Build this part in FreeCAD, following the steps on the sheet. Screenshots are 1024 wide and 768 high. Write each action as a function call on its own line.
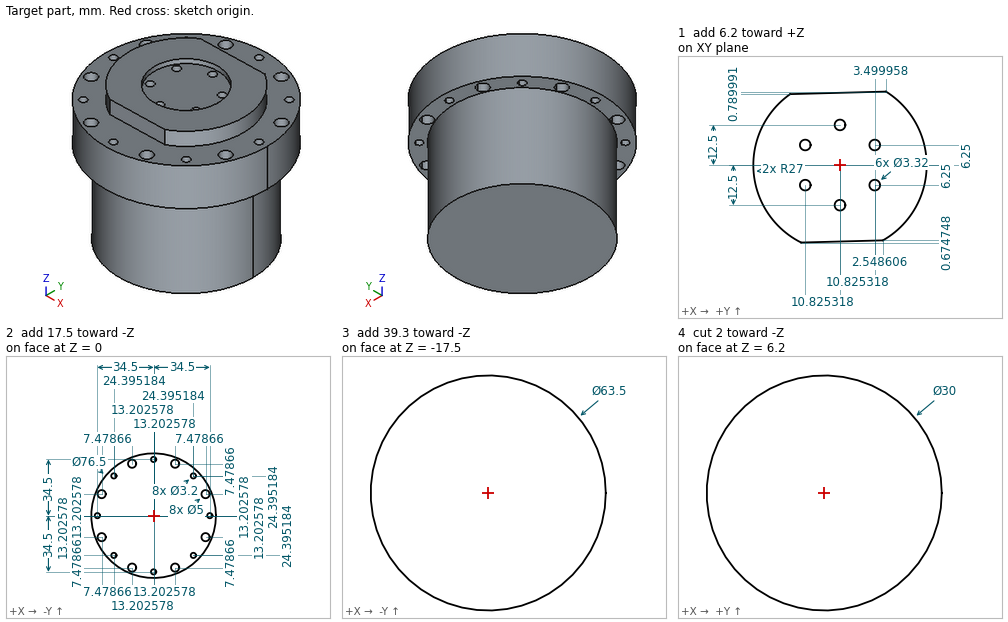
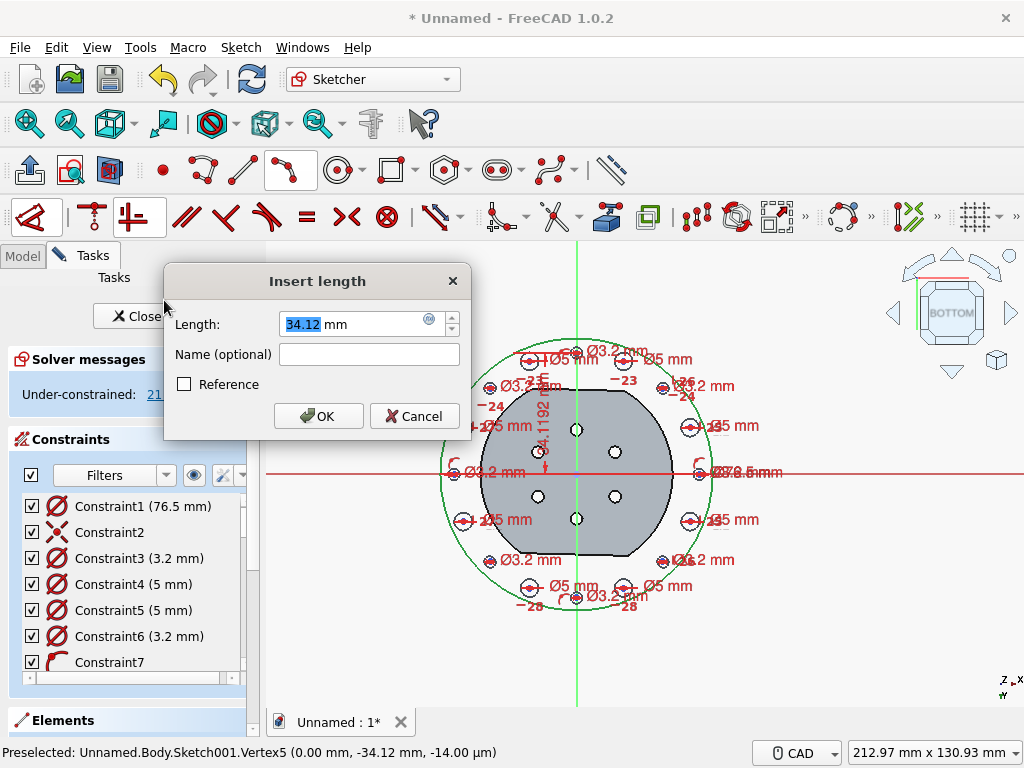
text(34.5)
key(Return)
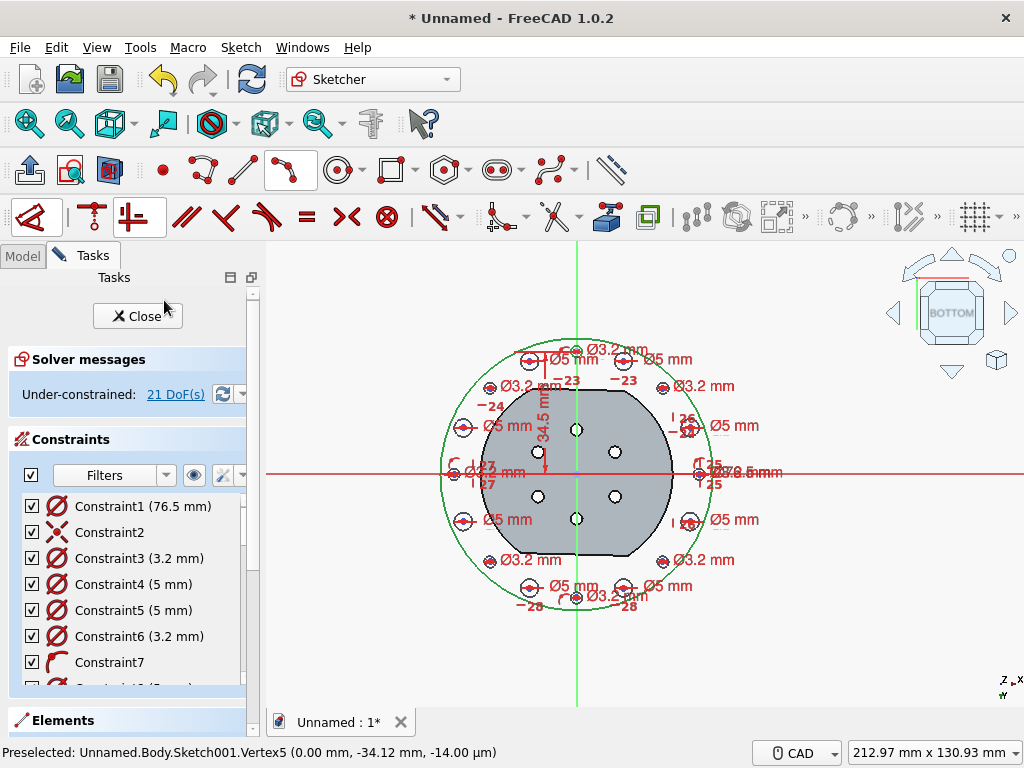
click(699, 474)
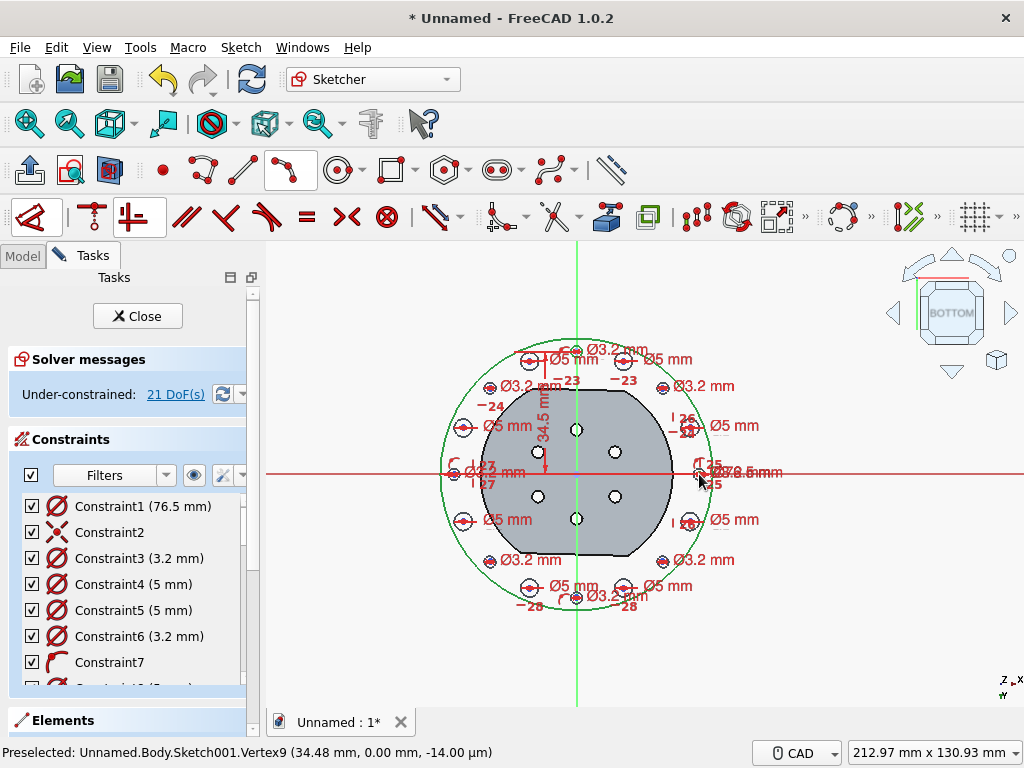
key(l)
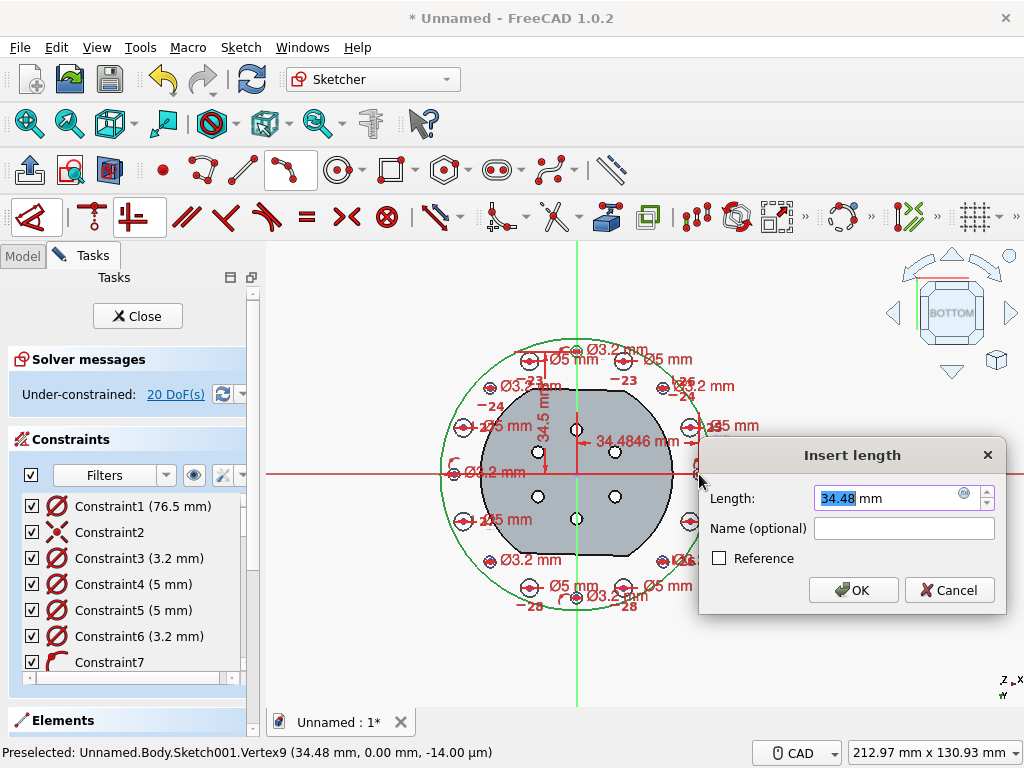
text(34.5)
key(Return)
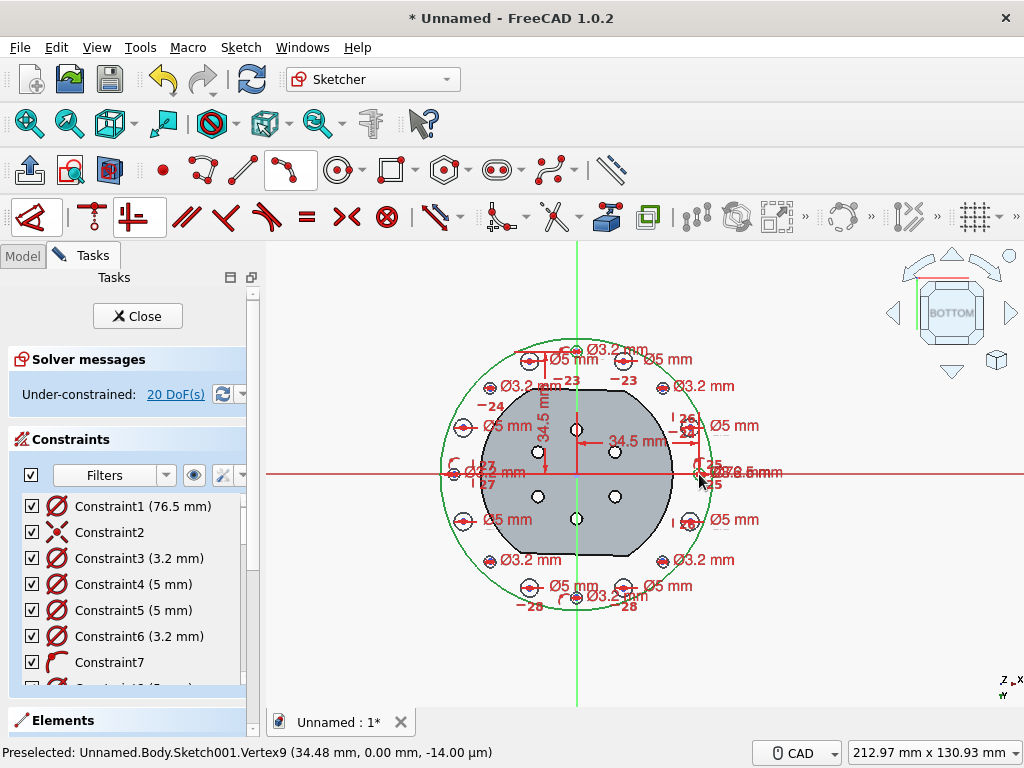
click(454, 474)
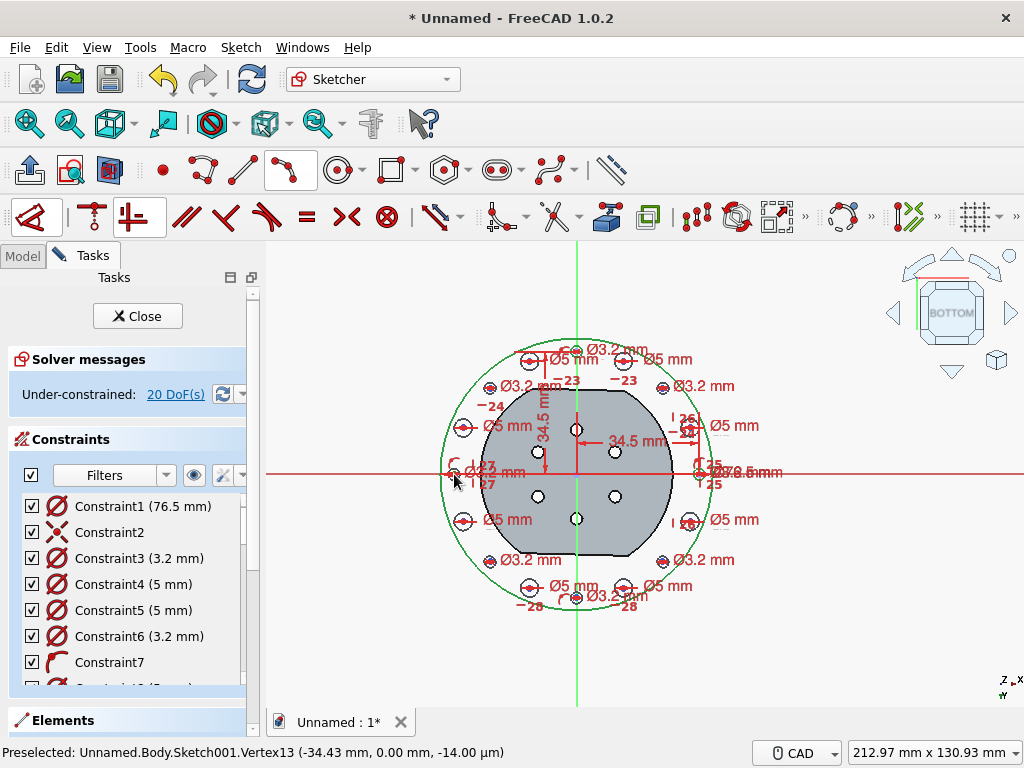
key(l)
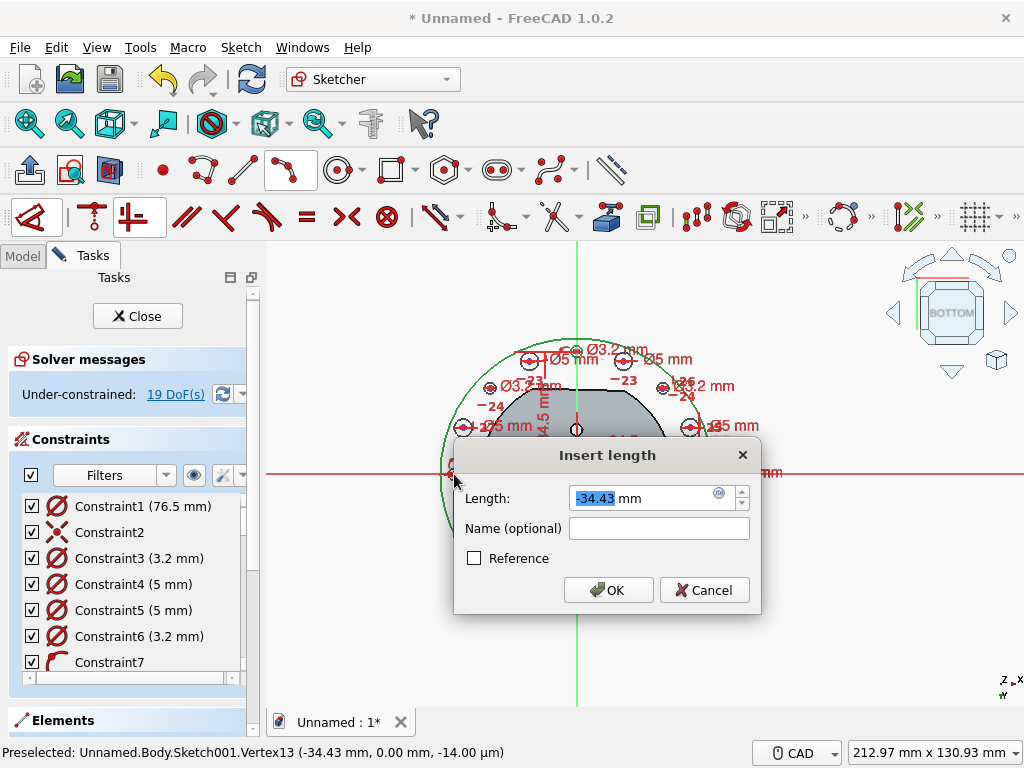
text(-34.5)
key(Return)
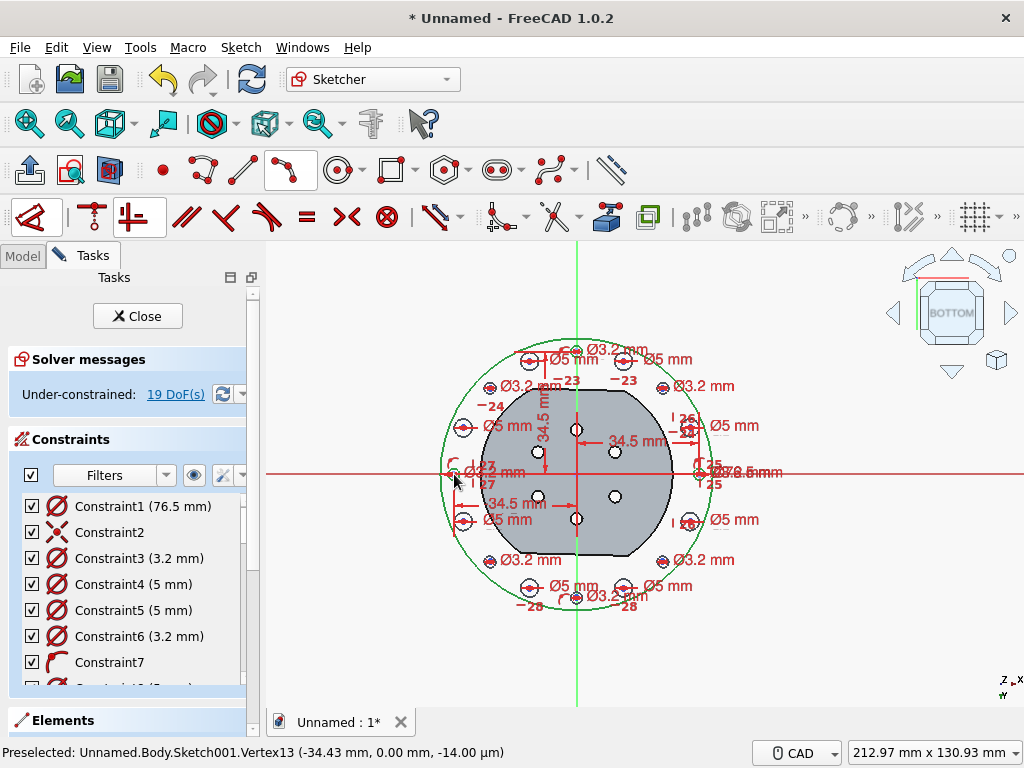
click(577, 598)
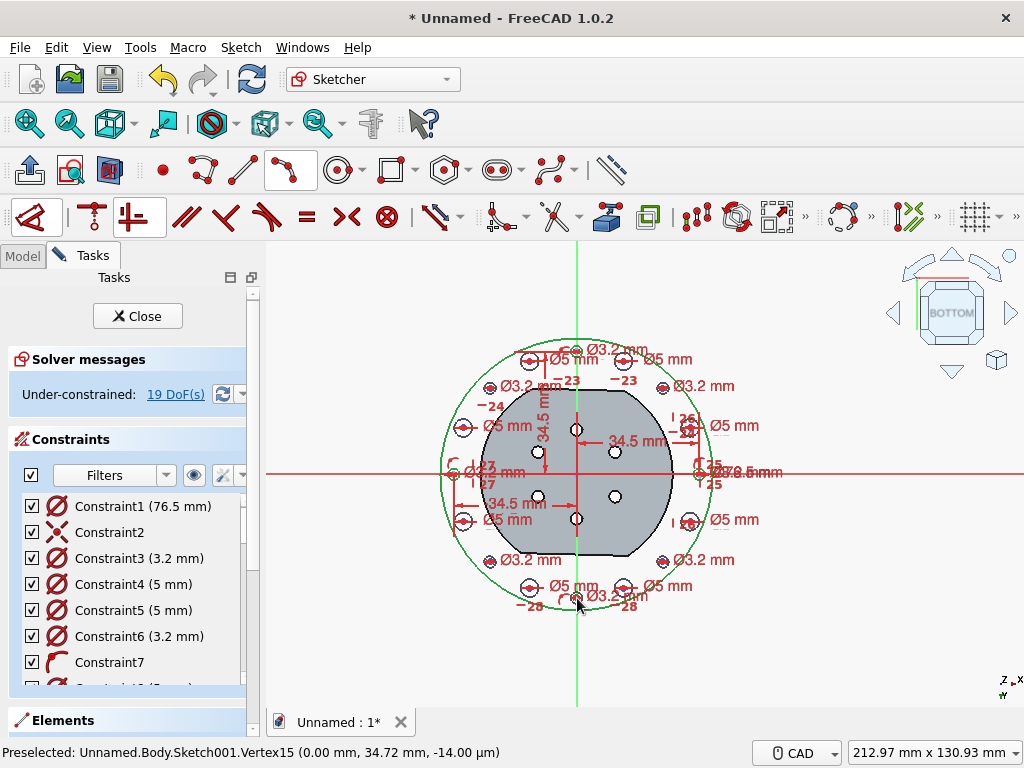
key(i)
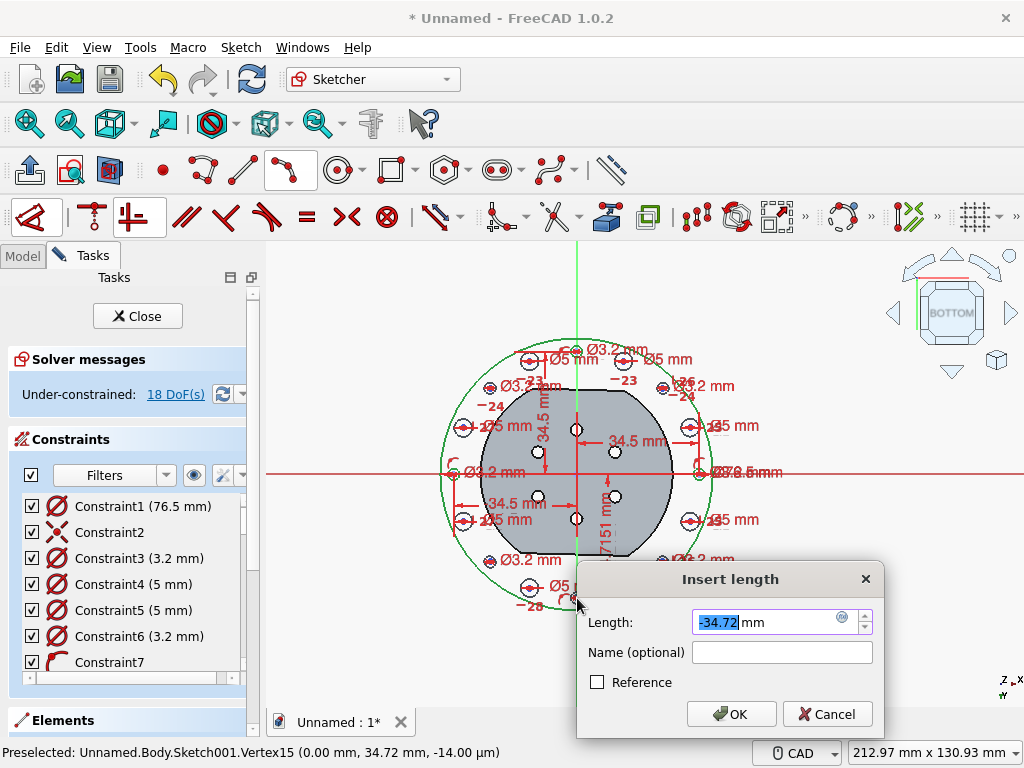
text(-34.5)
key(Return)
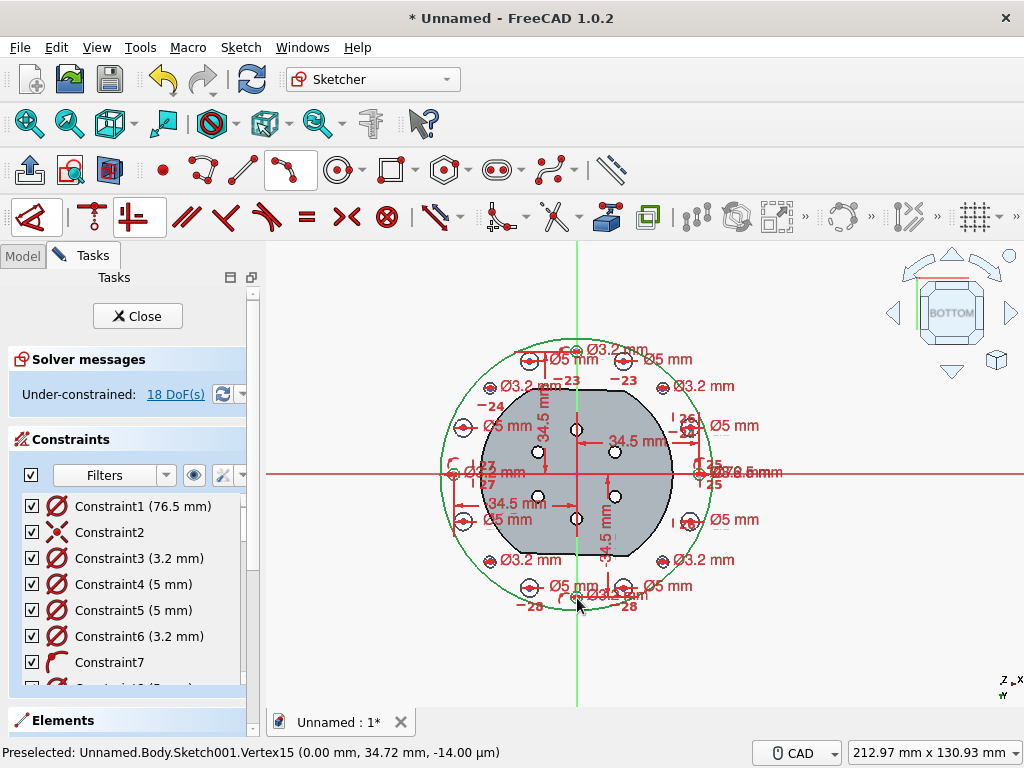
scroll(663, 388, up, 2)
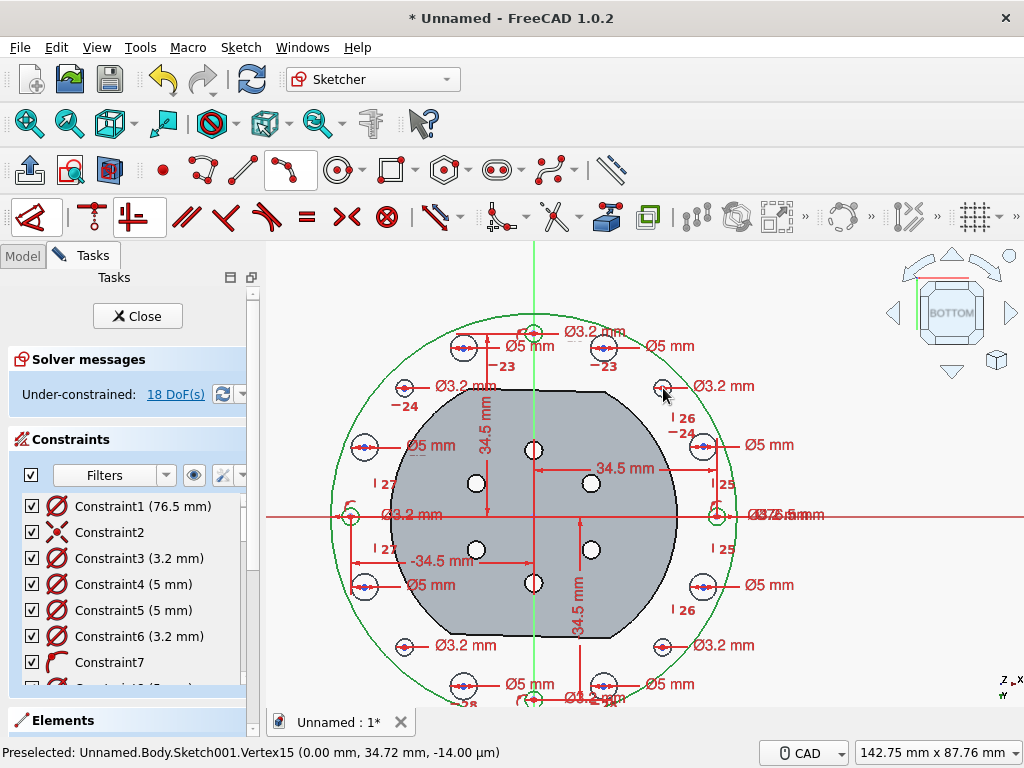
click(663, 388)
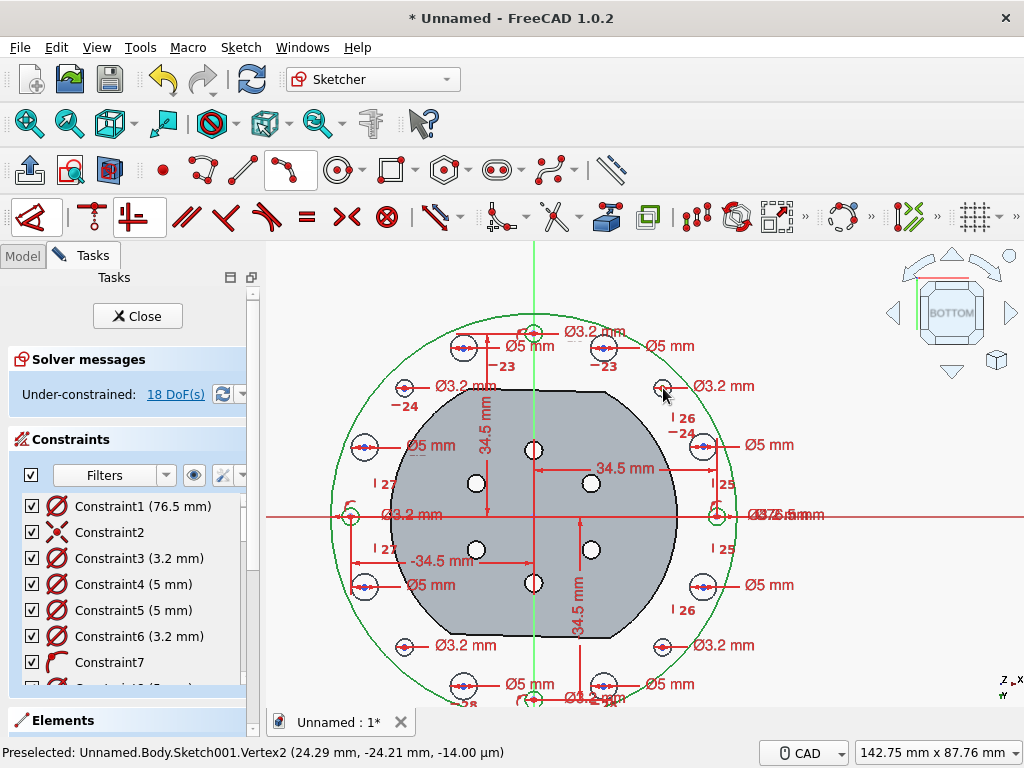
click(604, 348)